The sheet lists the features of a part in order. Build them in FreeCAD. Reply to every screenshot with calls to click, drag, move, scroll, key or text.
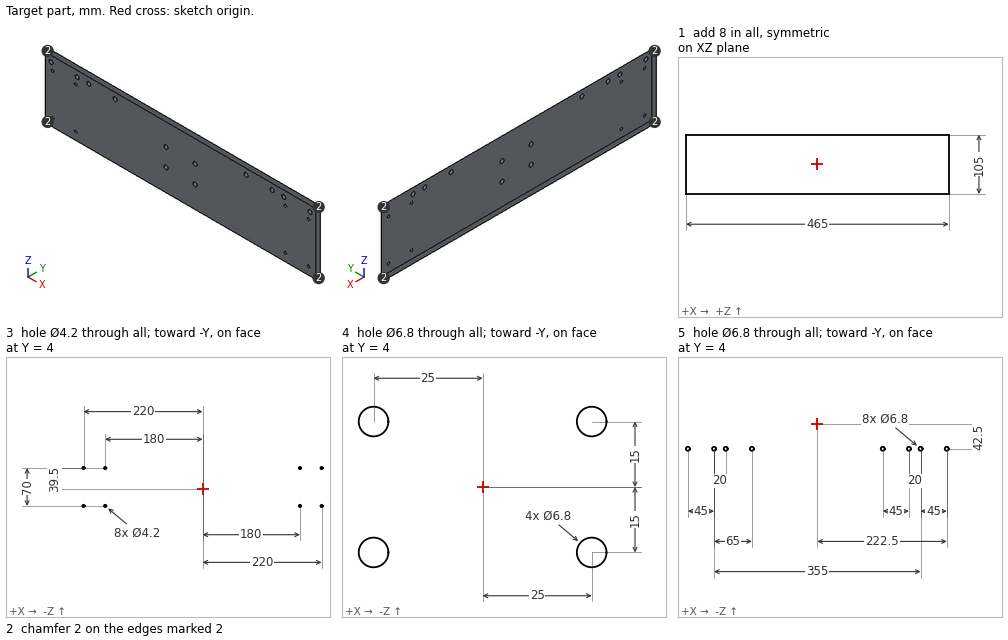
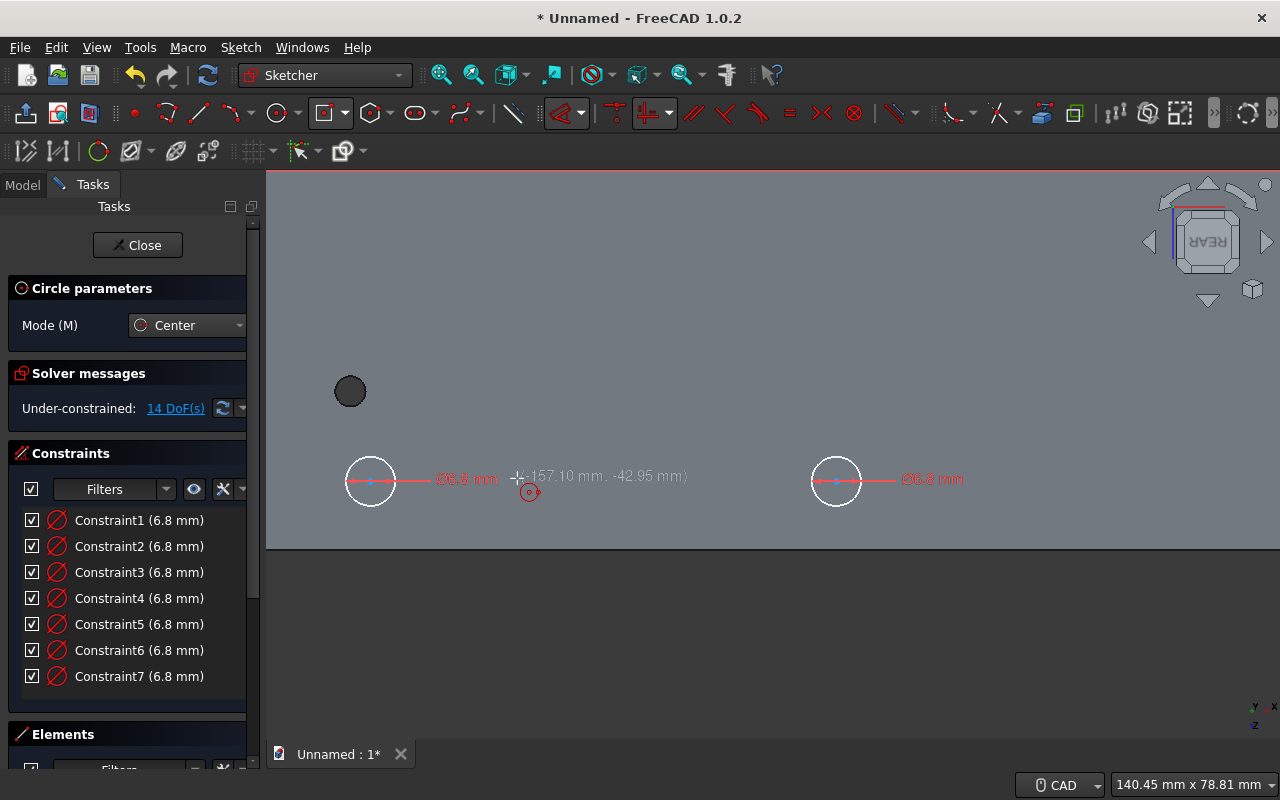
scroll(517, 478, down, 9)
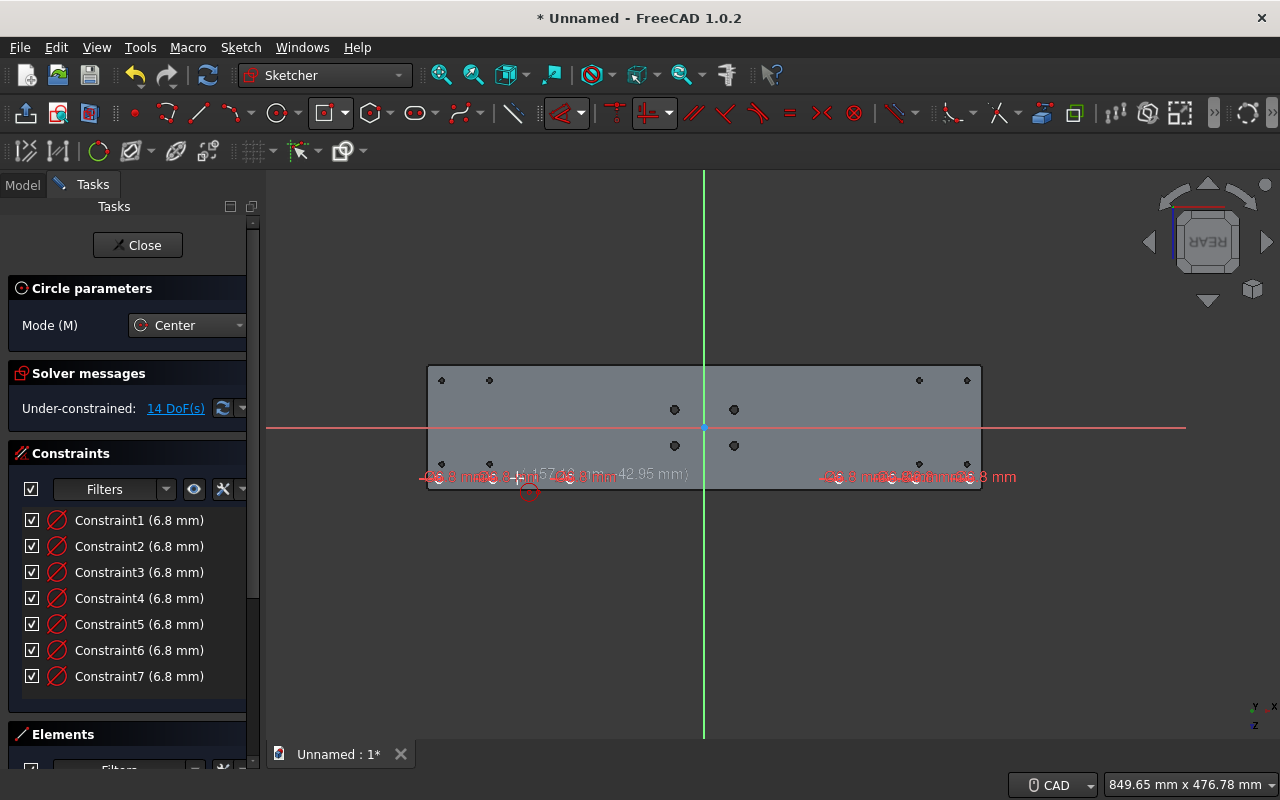
click(517, 478)
move(519, 476)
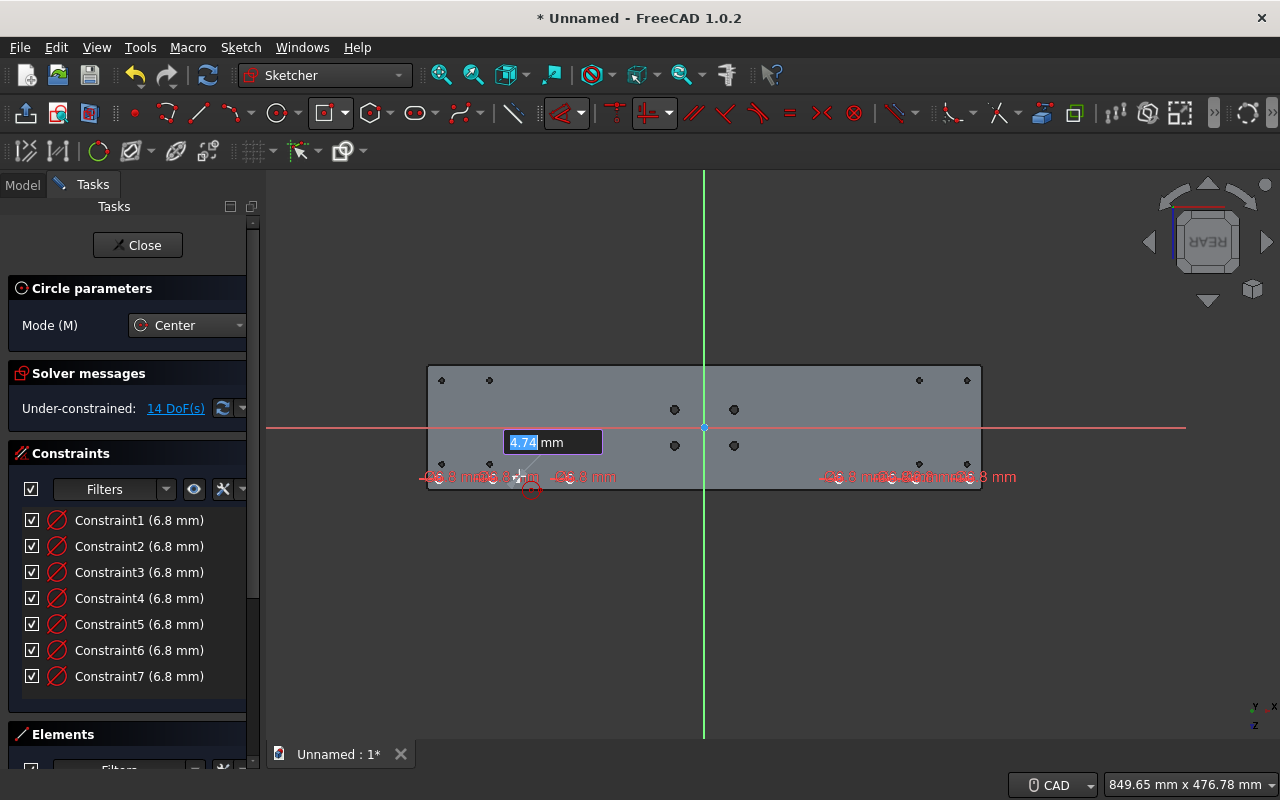
text(6.8)
key(Return)
key(Escape)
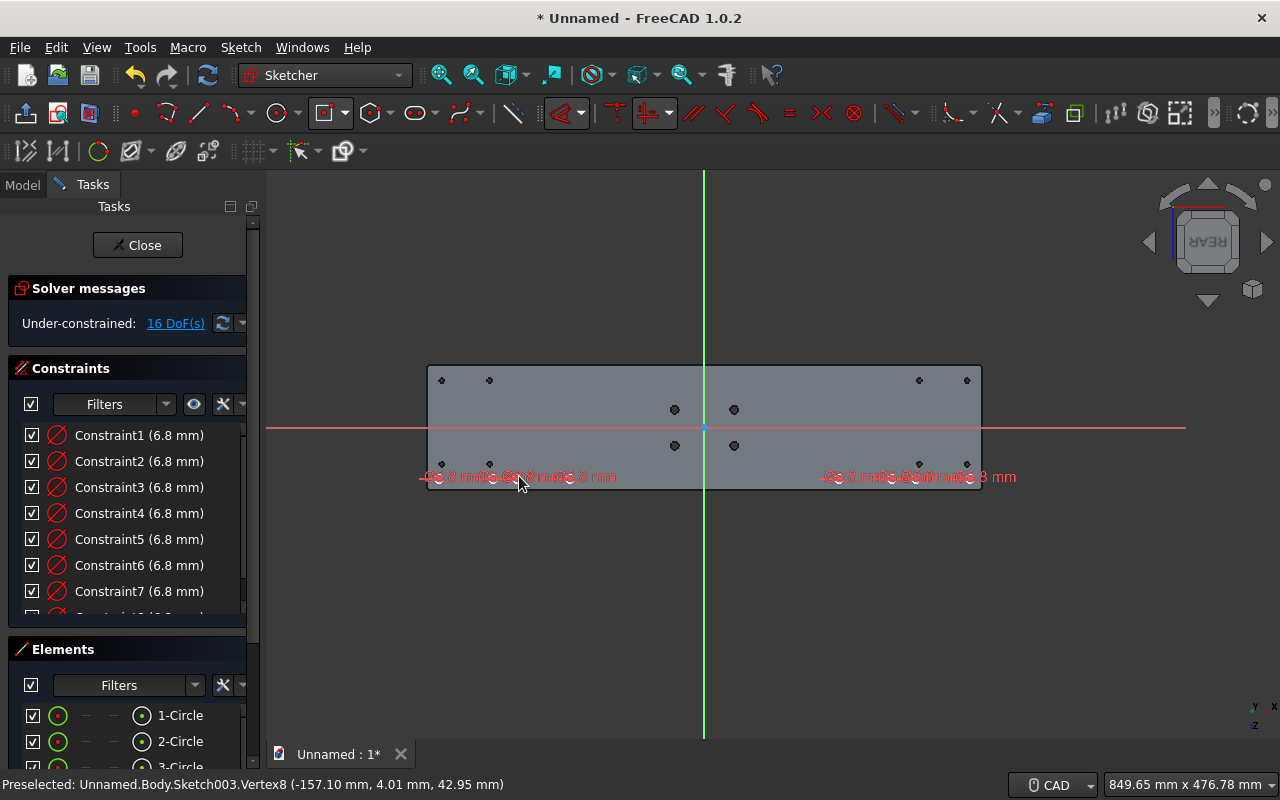
click(970, 479)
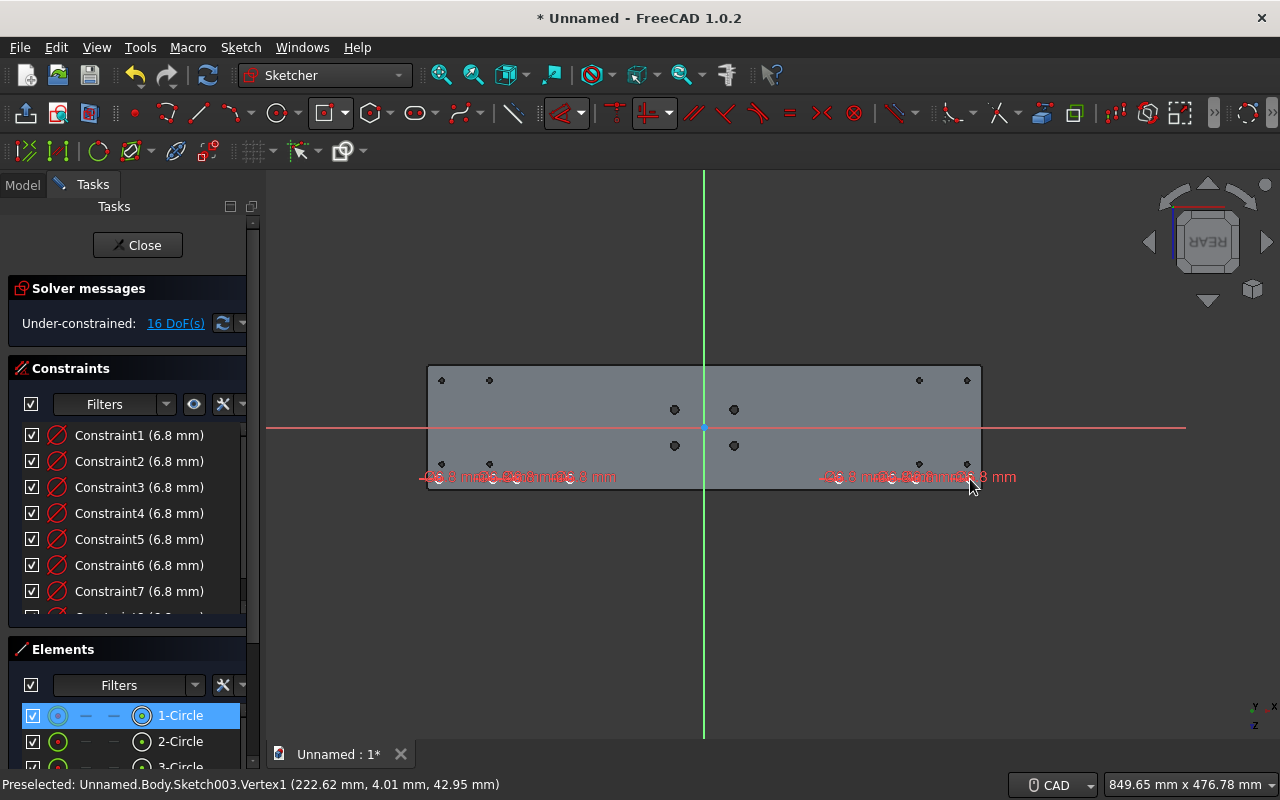
click(916, 479)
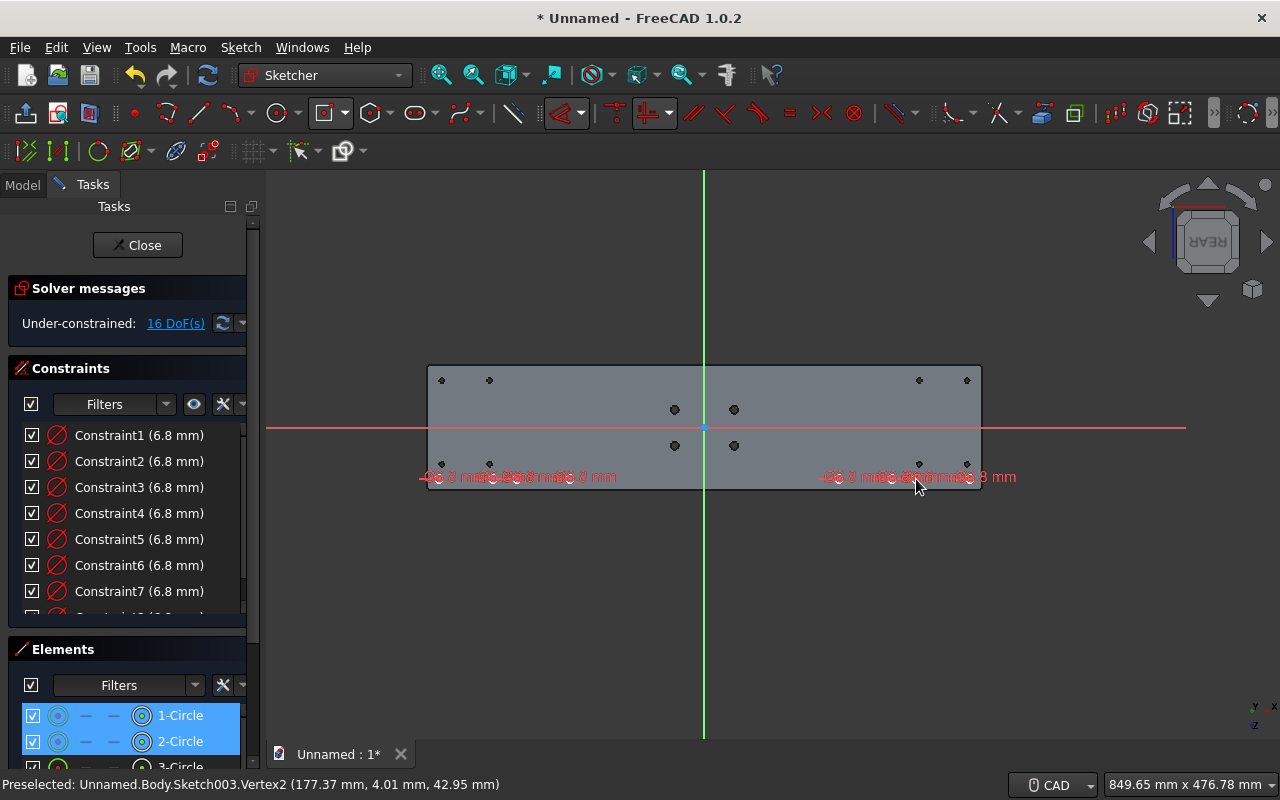
click(672, 114)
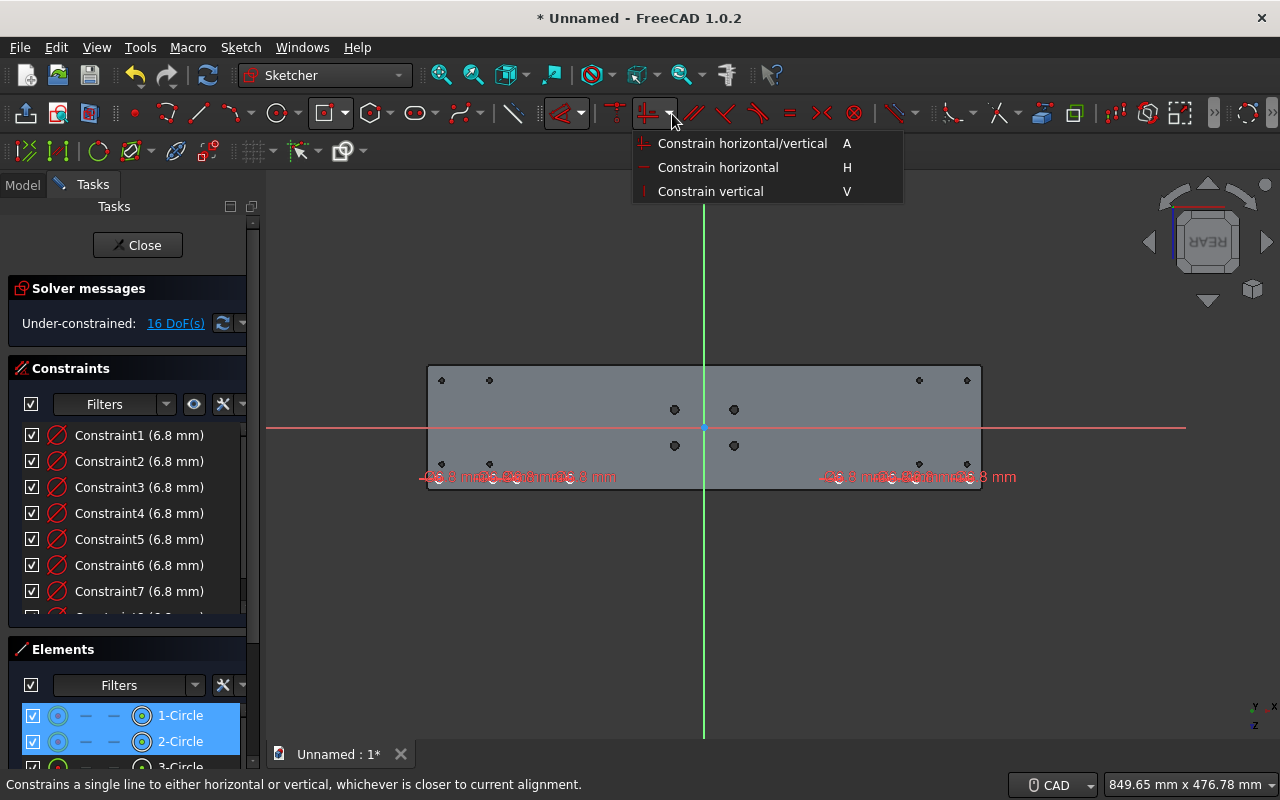
click(768, 167)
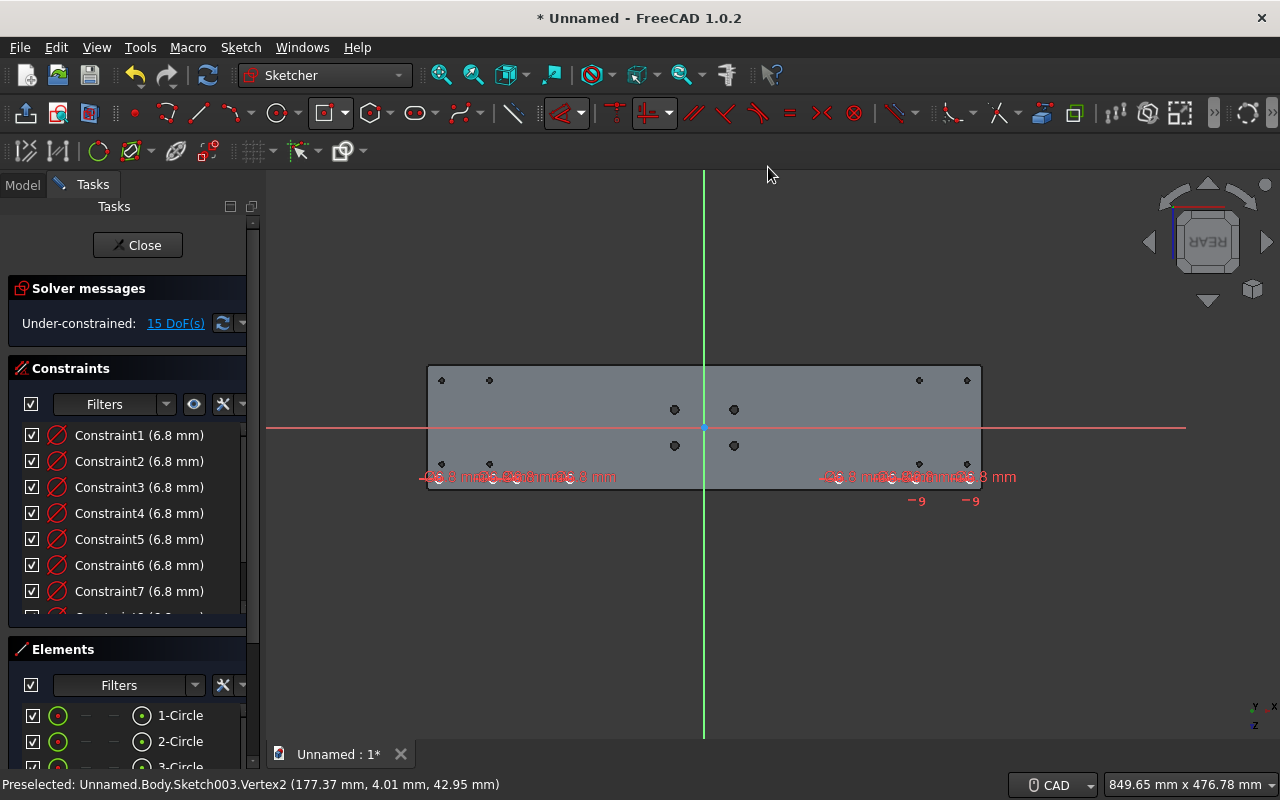
click(916, 479)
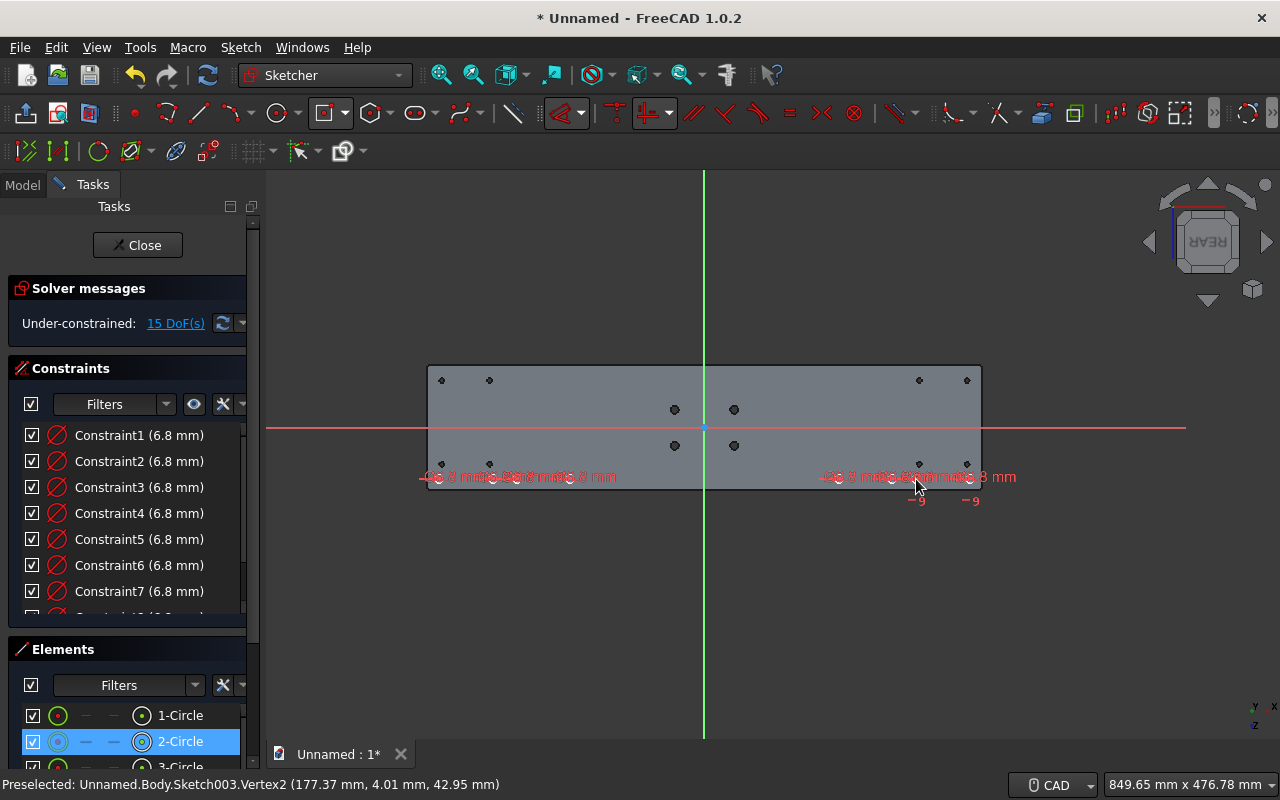
click(493, 479)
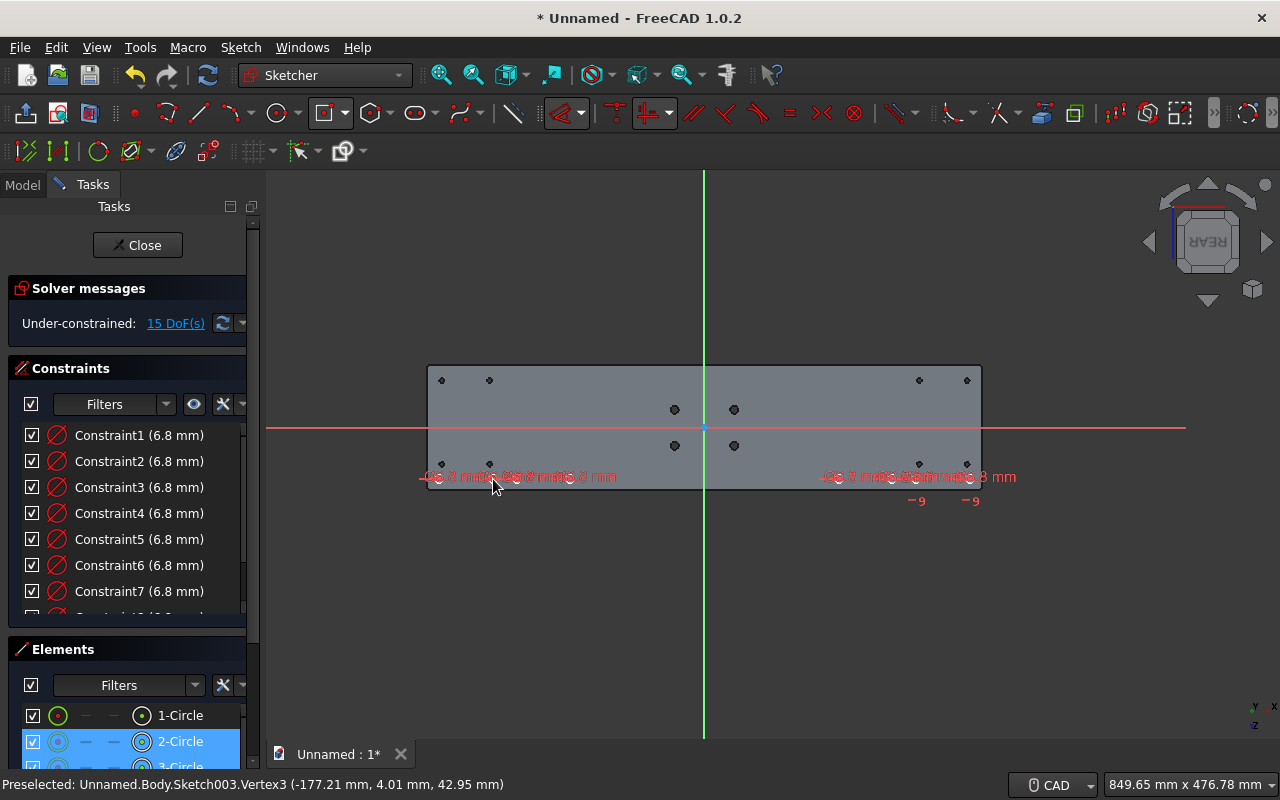
click(672, 114)